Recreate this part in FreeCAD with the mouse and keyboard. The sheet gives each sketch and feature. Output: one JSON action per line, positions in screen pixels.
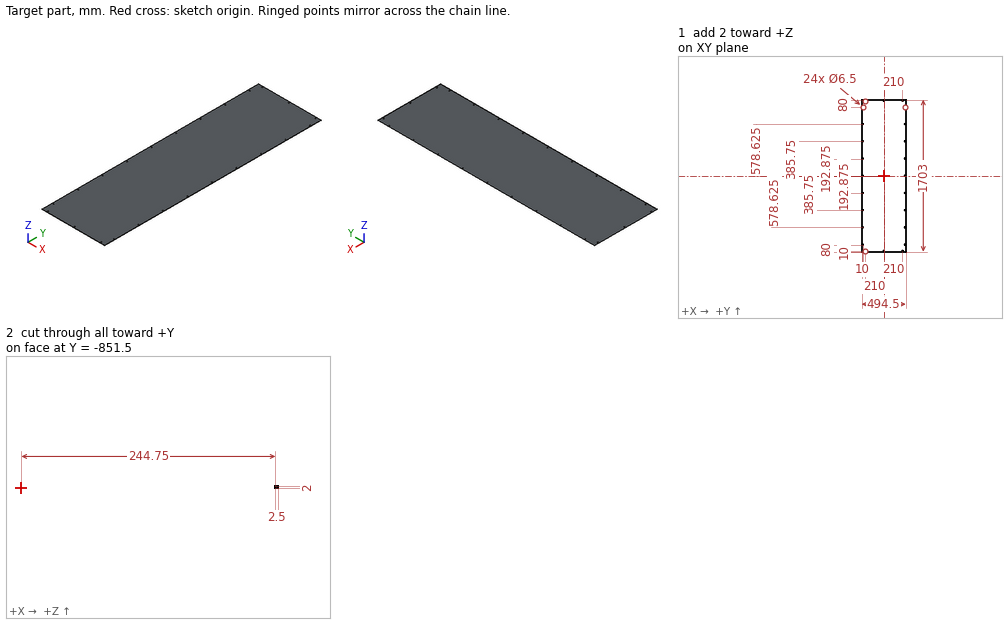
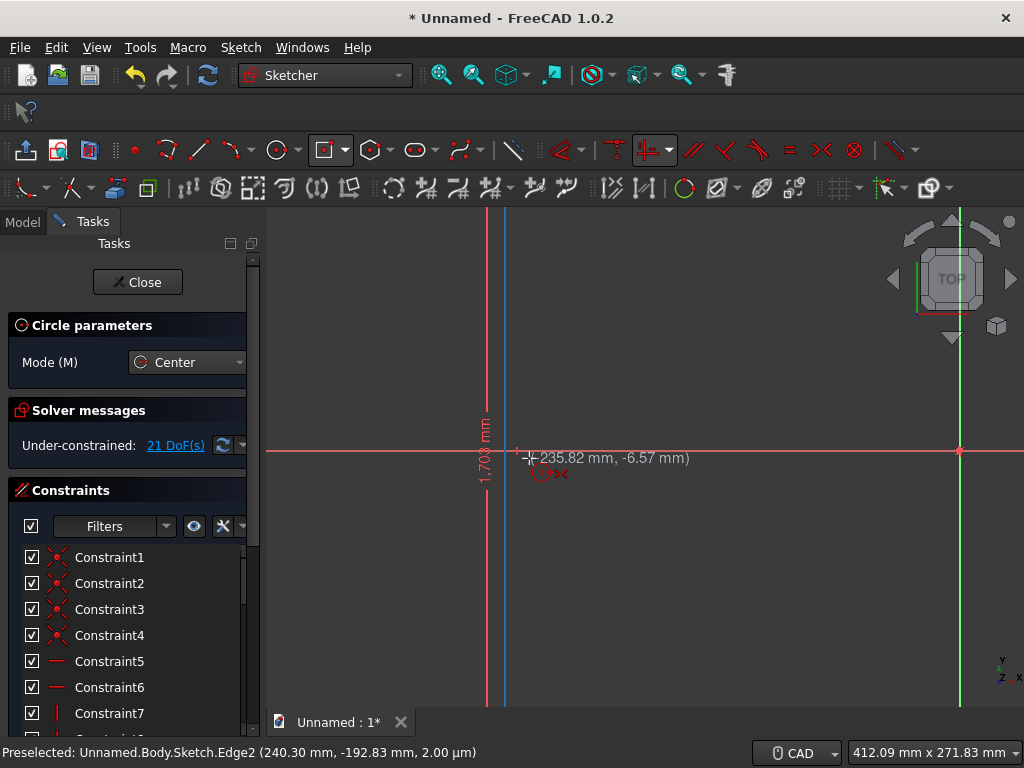
{"action": "left_click", "coordinate": [524, 451]}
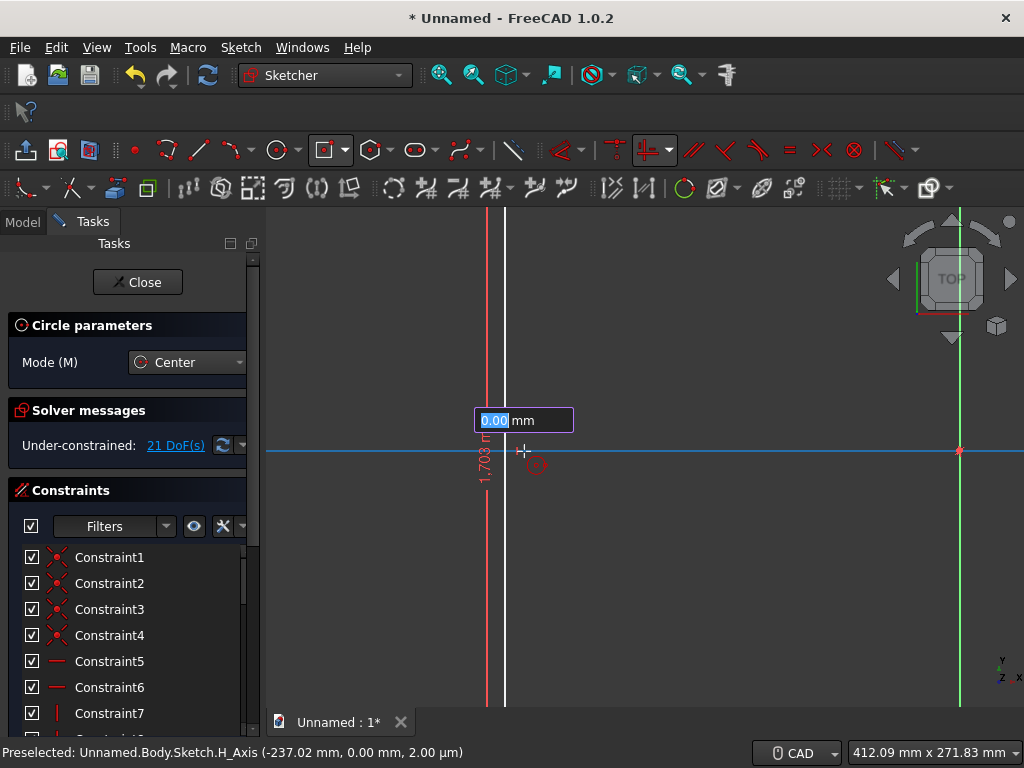
{"action": "scroll", "coordinate": [522, 457], "scroll_direction": "up", "scroll_amount": 6}
{"action": "mouse_move", "coordinate": [520, 454]}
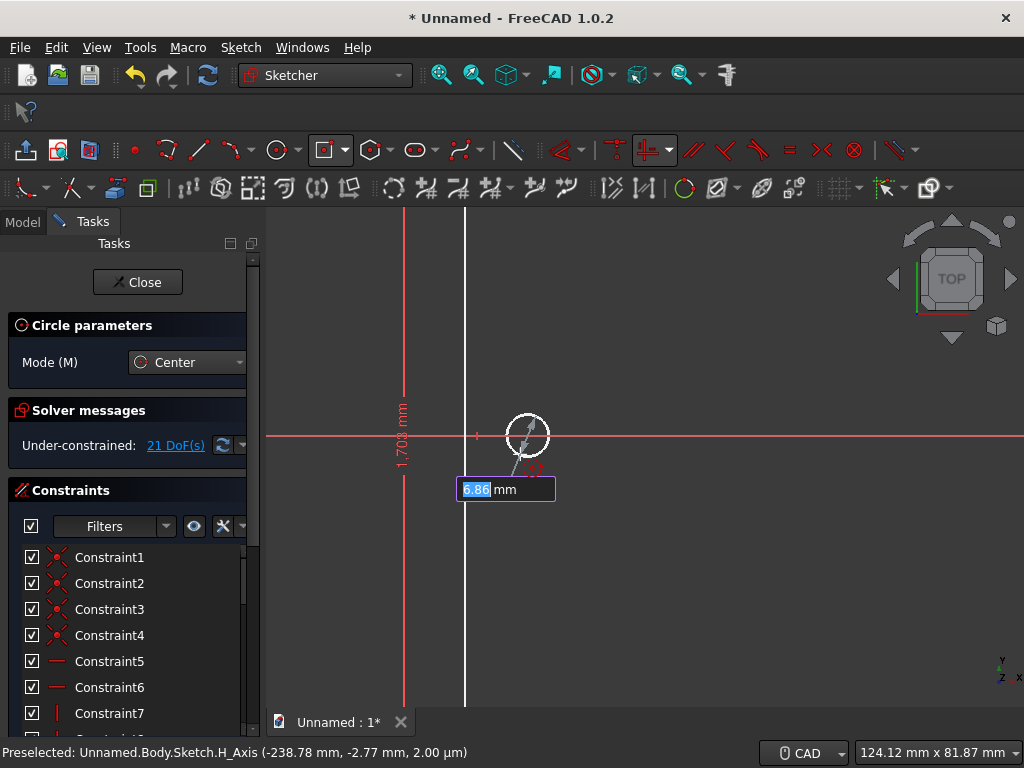
{"action": "type", "text": "6.5"}
{"action": "key", "text": "Return"}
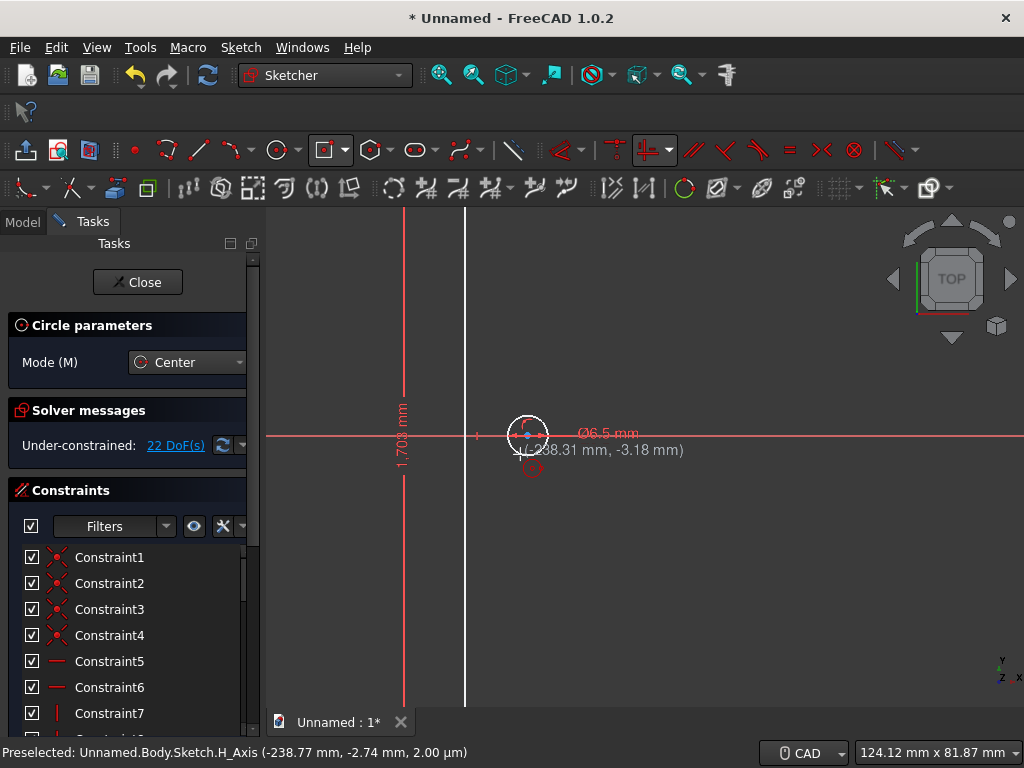
{"action": "scroll", "coordinate": [528, 458], "scroll_direction": "down", "scroll_amount": 17}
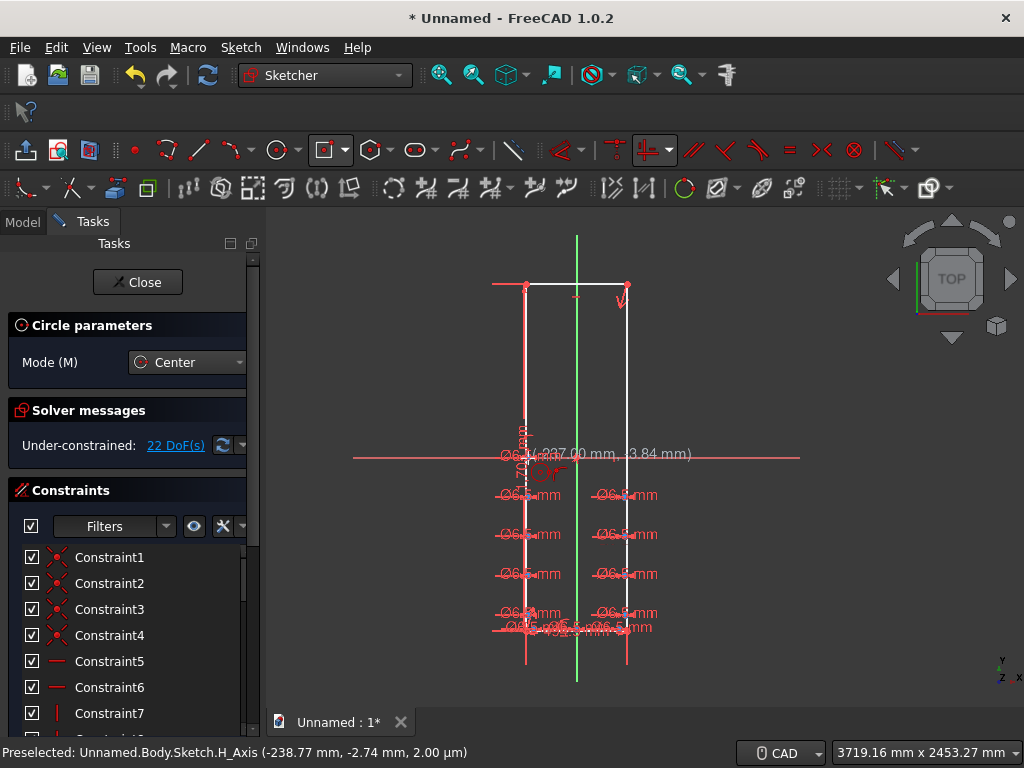
{"action": "scroll", "coordinate": [528, 418], "scroll_direction": "up", "scroll_amount": 18}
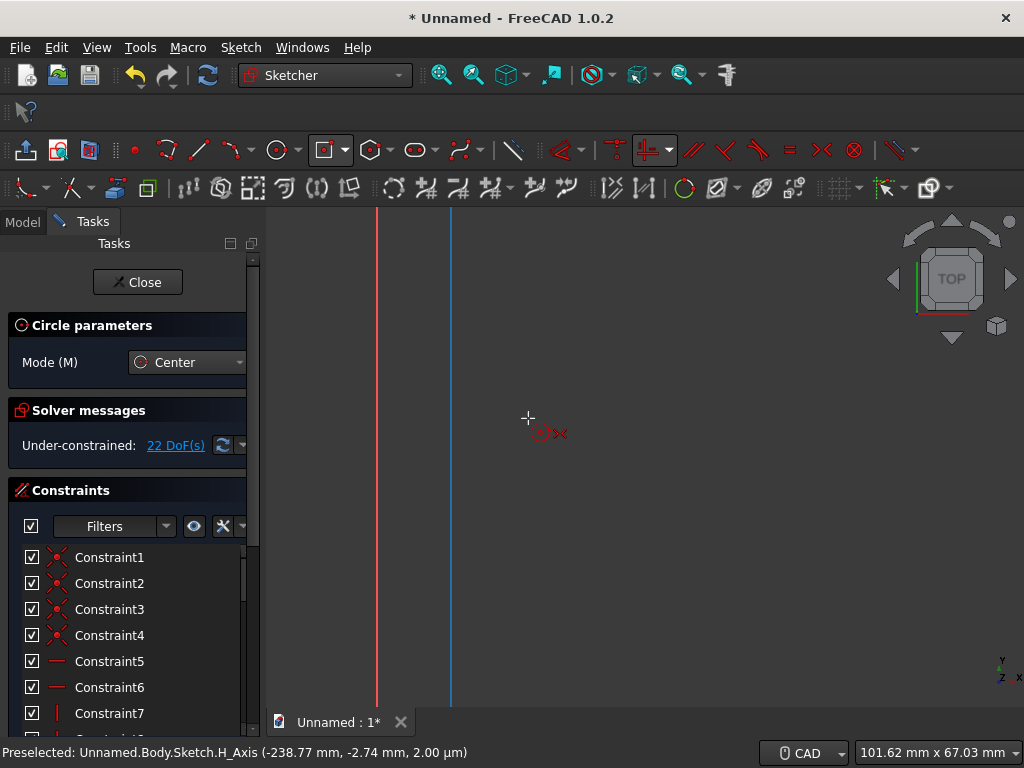
{"action": "scroll", "coordinate": [528, 418], "scroll_direction": "down", "scroll_amount": 18}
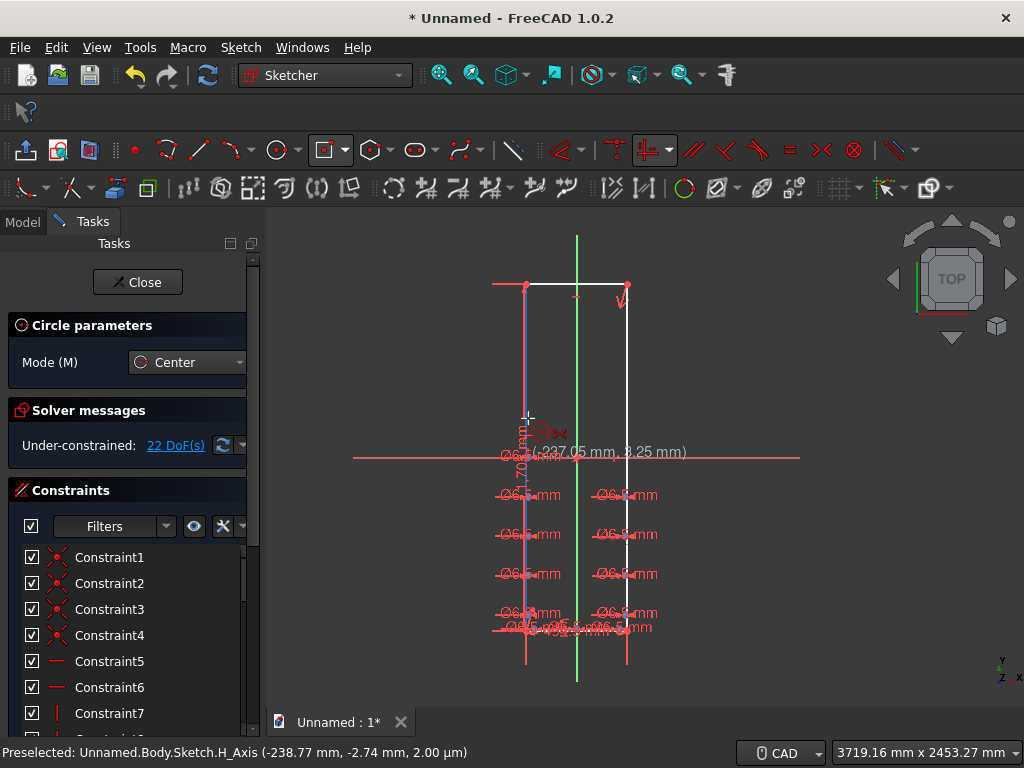
{"action": "scroll", "coordinate": [528, 418], "scroll_direction": "up", "scroll_amount": 11}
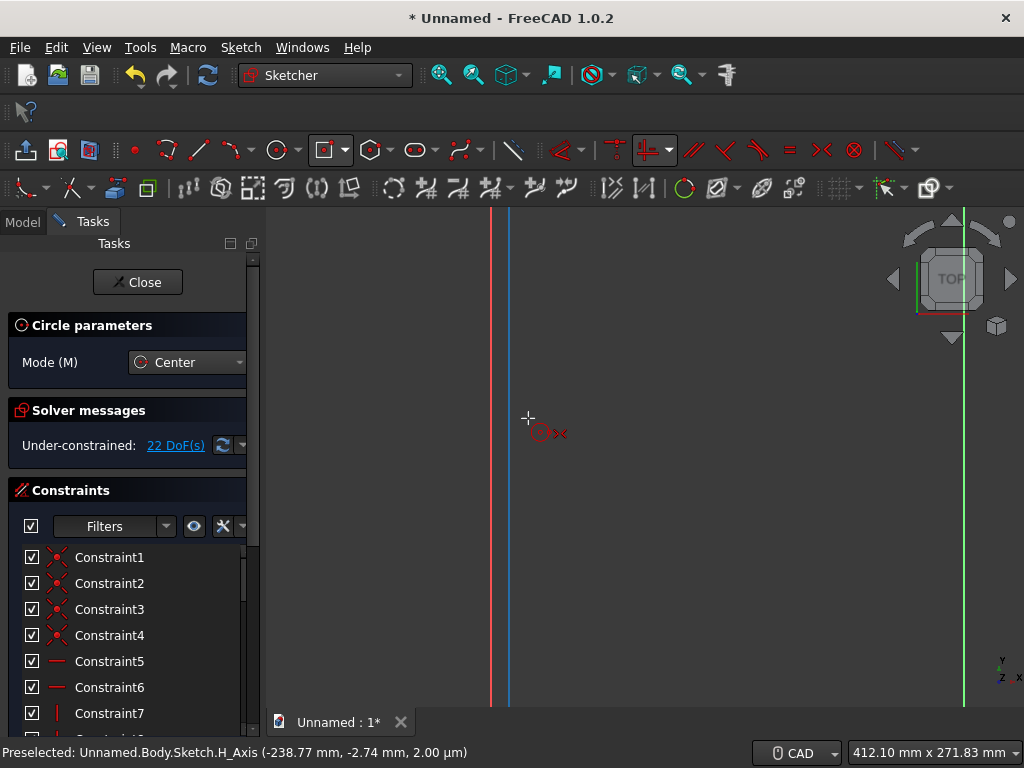
{"action": "left_click", "coordinate": [528, 418]}
{"action": "mouse_move", "coordinate": [532, 414]}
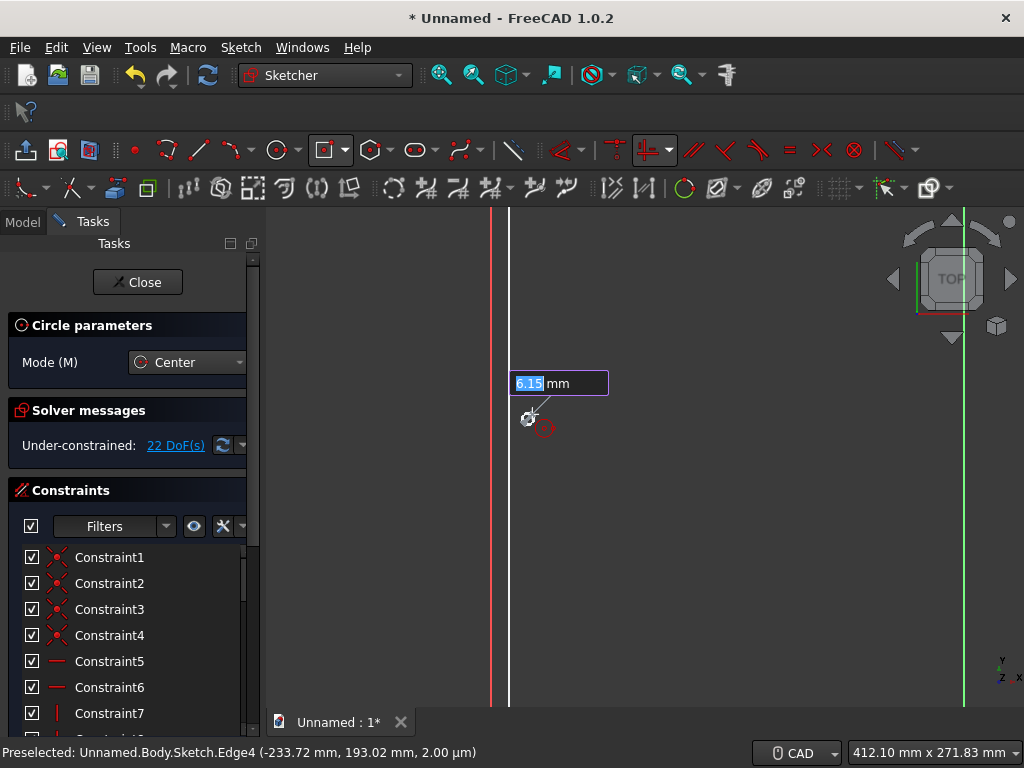
{"action": "type", "text": "6.5"}
{"action": "key", "text": "Return"}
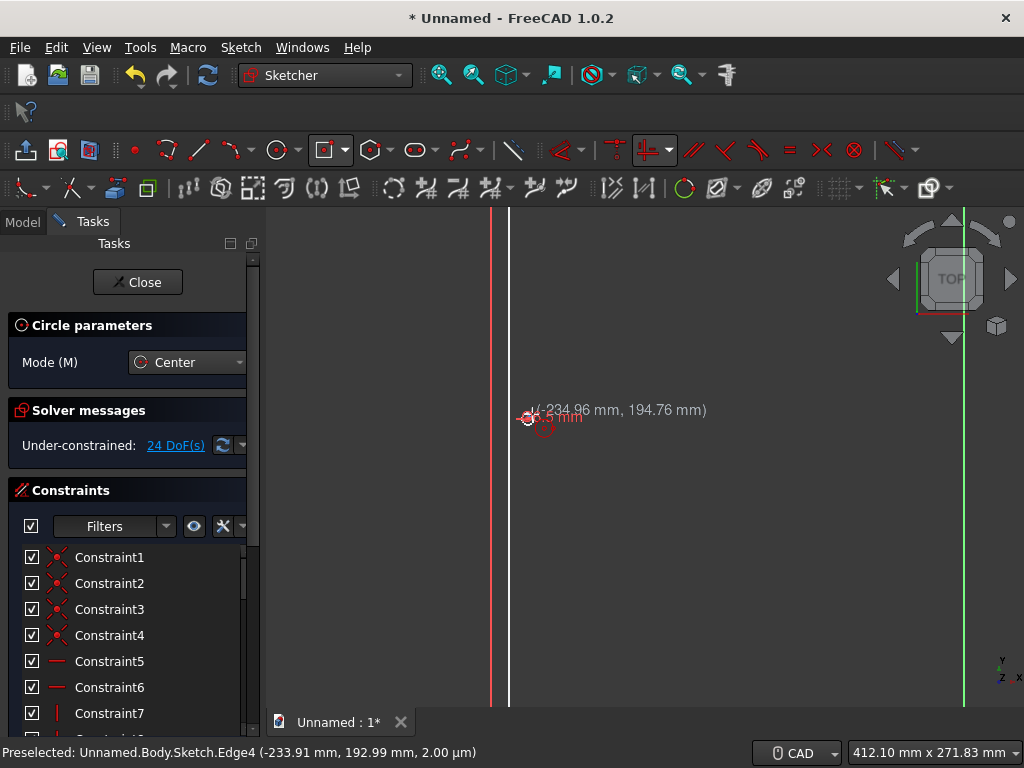
{"action": "scroll", "coordinate": [538, 425], "scroll_direction": "down", "scroll_amount": 12}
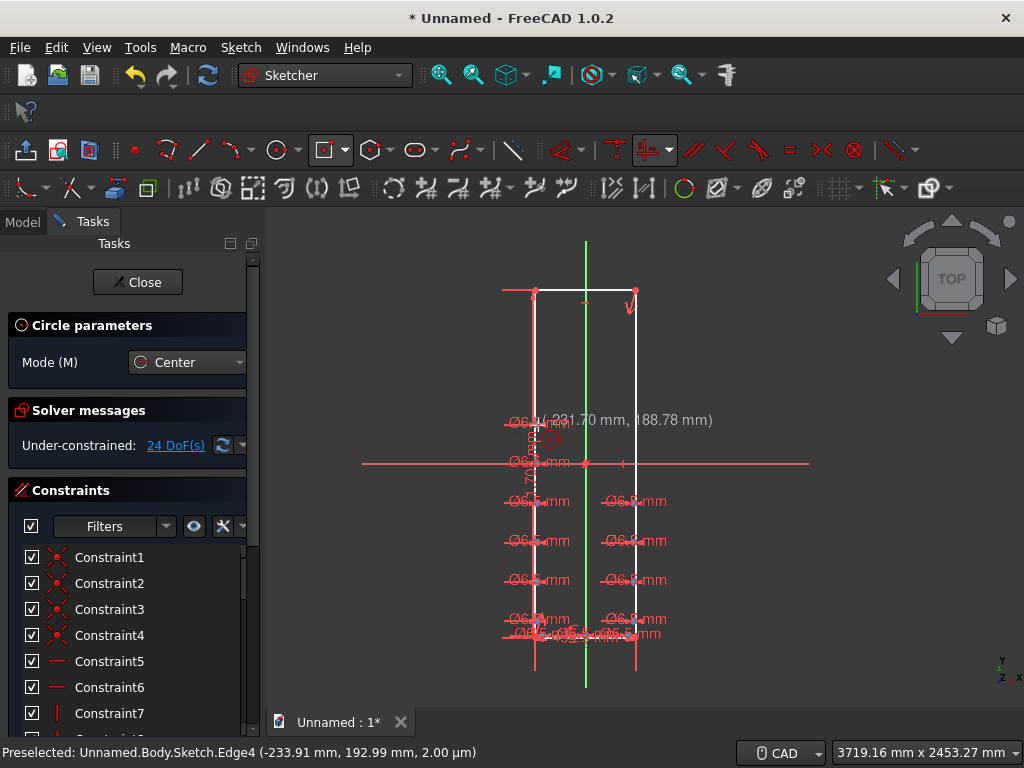
{"action": "scroll", "coordinate": [537, 393], "scroll_direction": "up", "scroll_amount": 19}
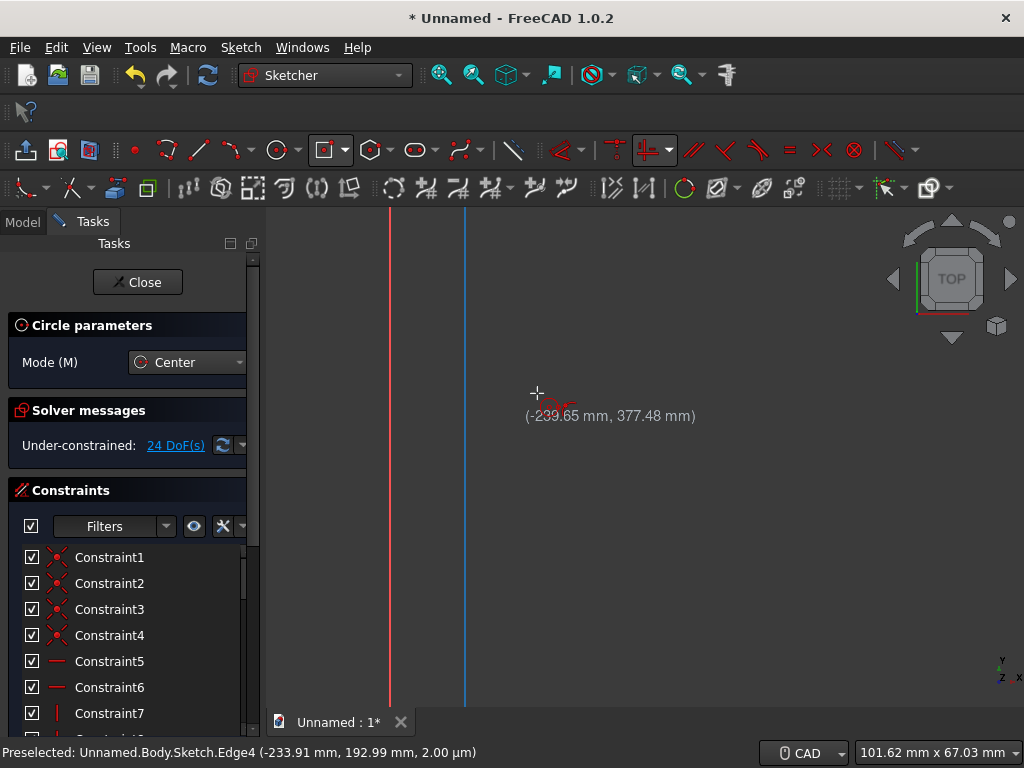
{"action": "scroll", "coordinate": [528, 379], "scroll_direction": "down", "scroll_amount": 18}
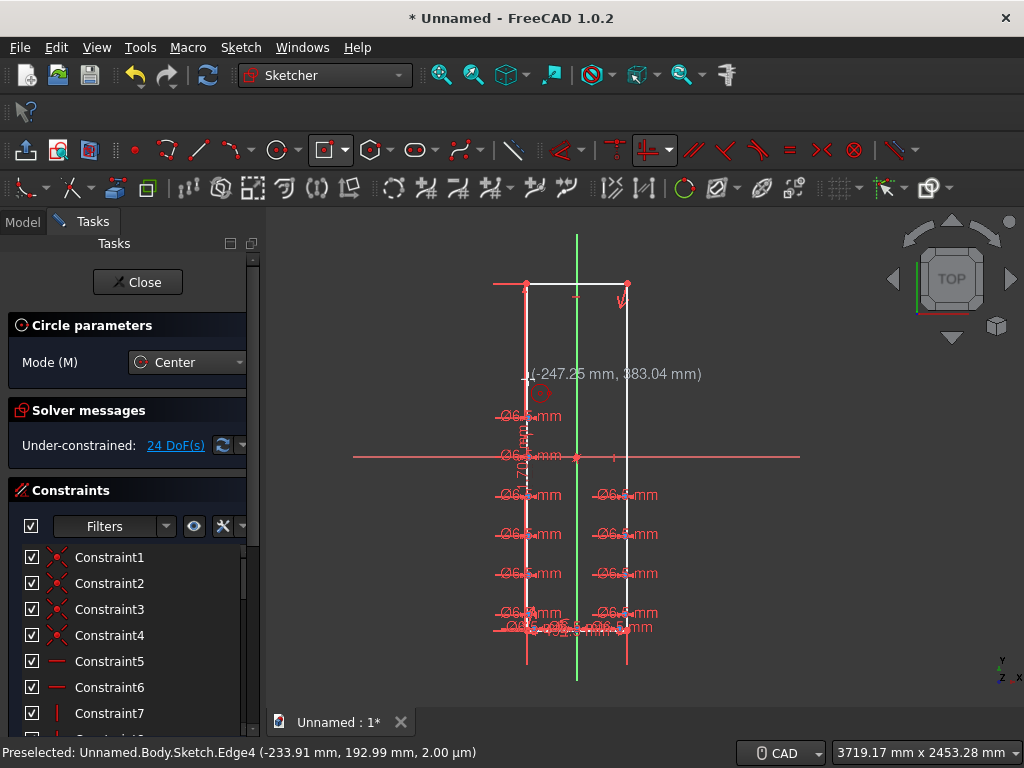
{"action": "scroll", "coordinate": [529, 379], "scroll_direction": "up", "scroll_amount": 11}